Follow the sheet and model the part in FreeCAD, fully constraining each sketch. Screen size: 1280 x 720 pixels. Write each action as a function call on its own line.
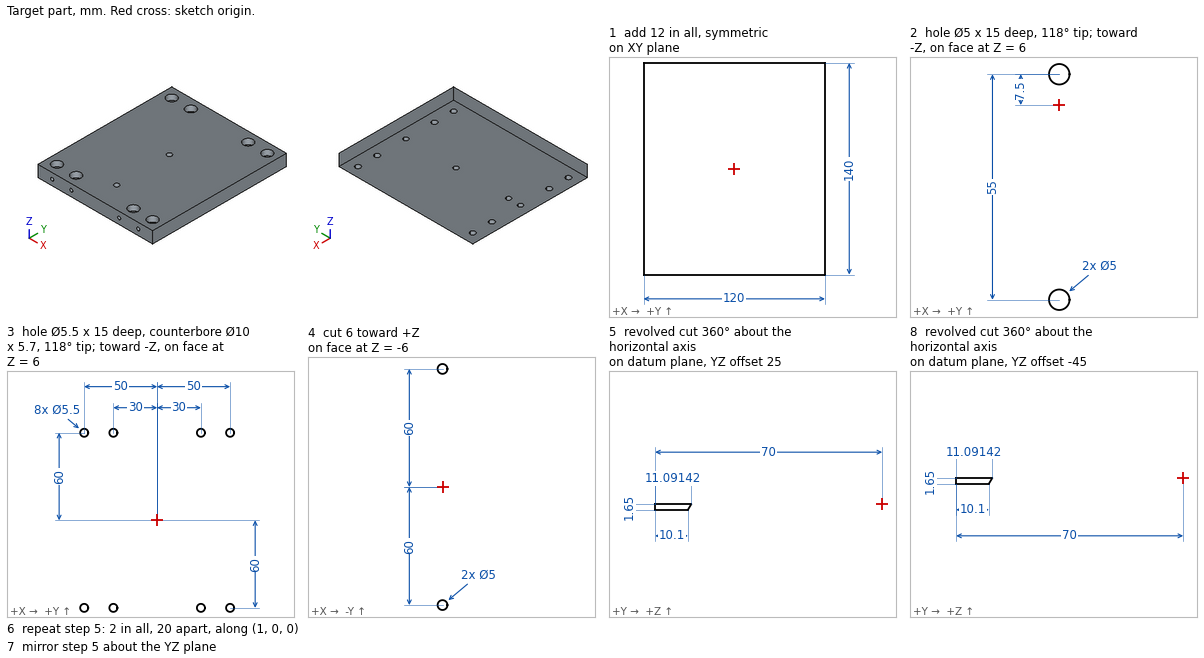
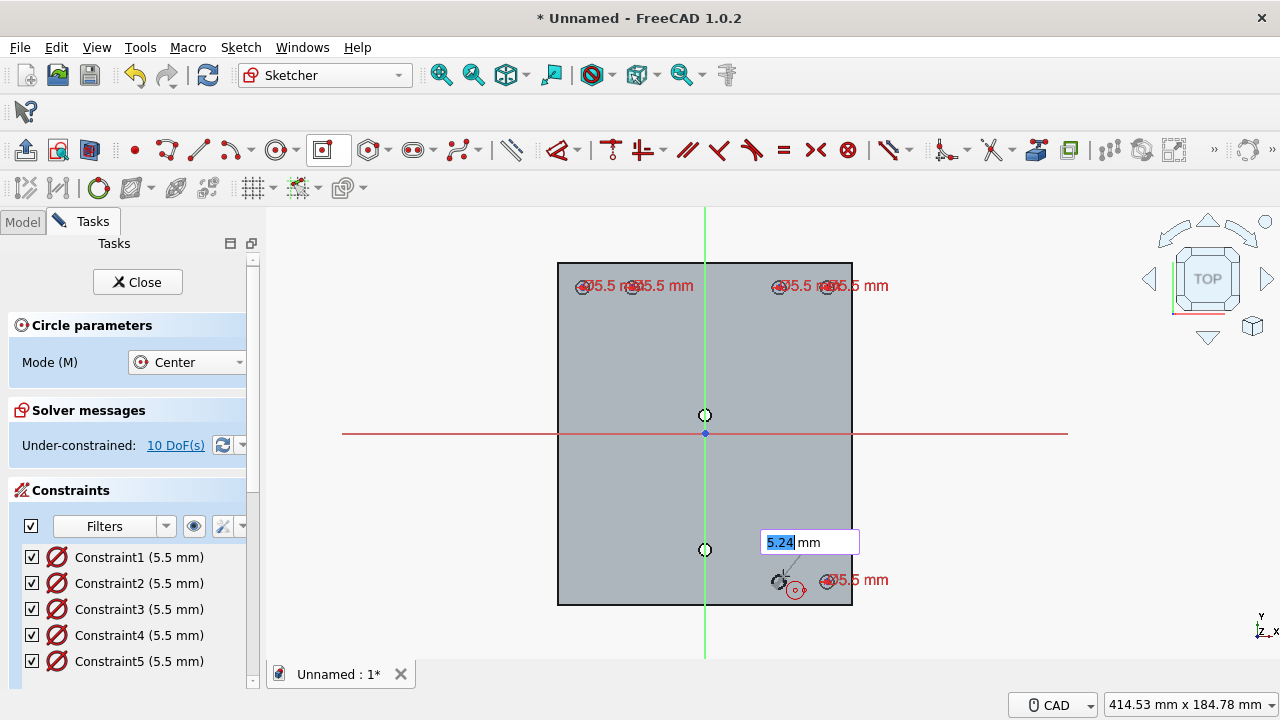
text(5.5)
key(Return)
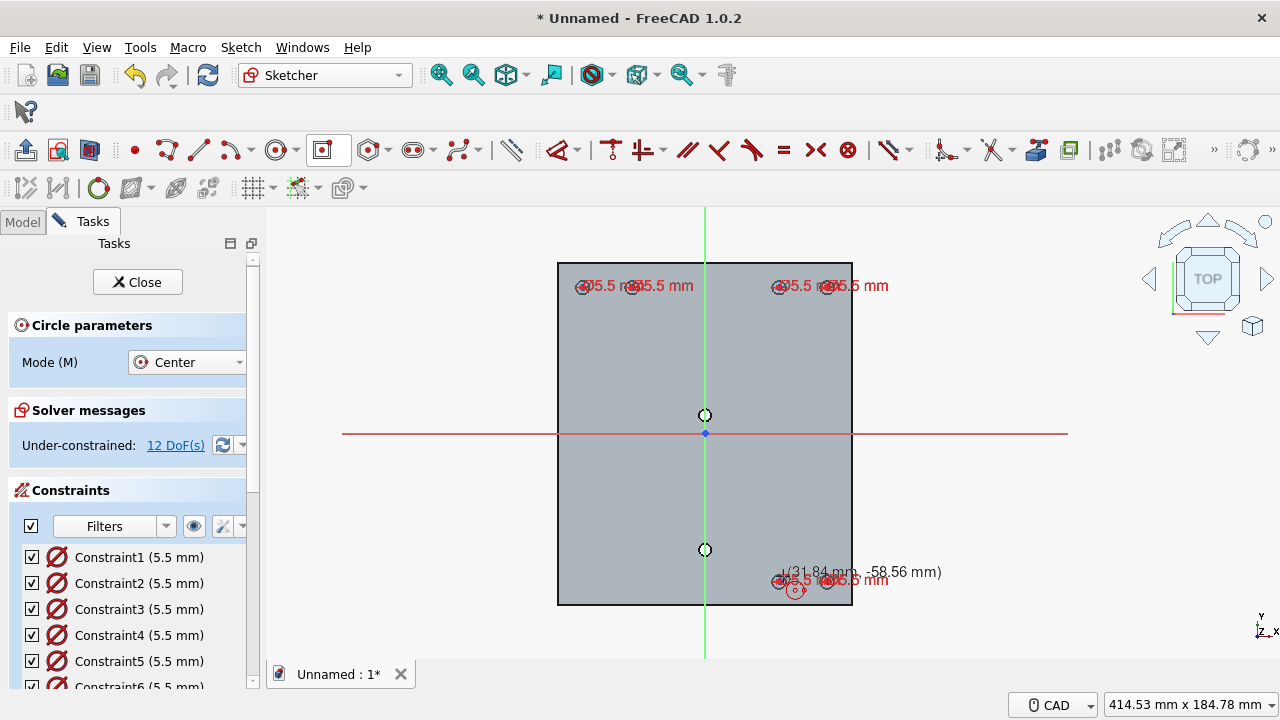
scroll(632, 581, up, 7)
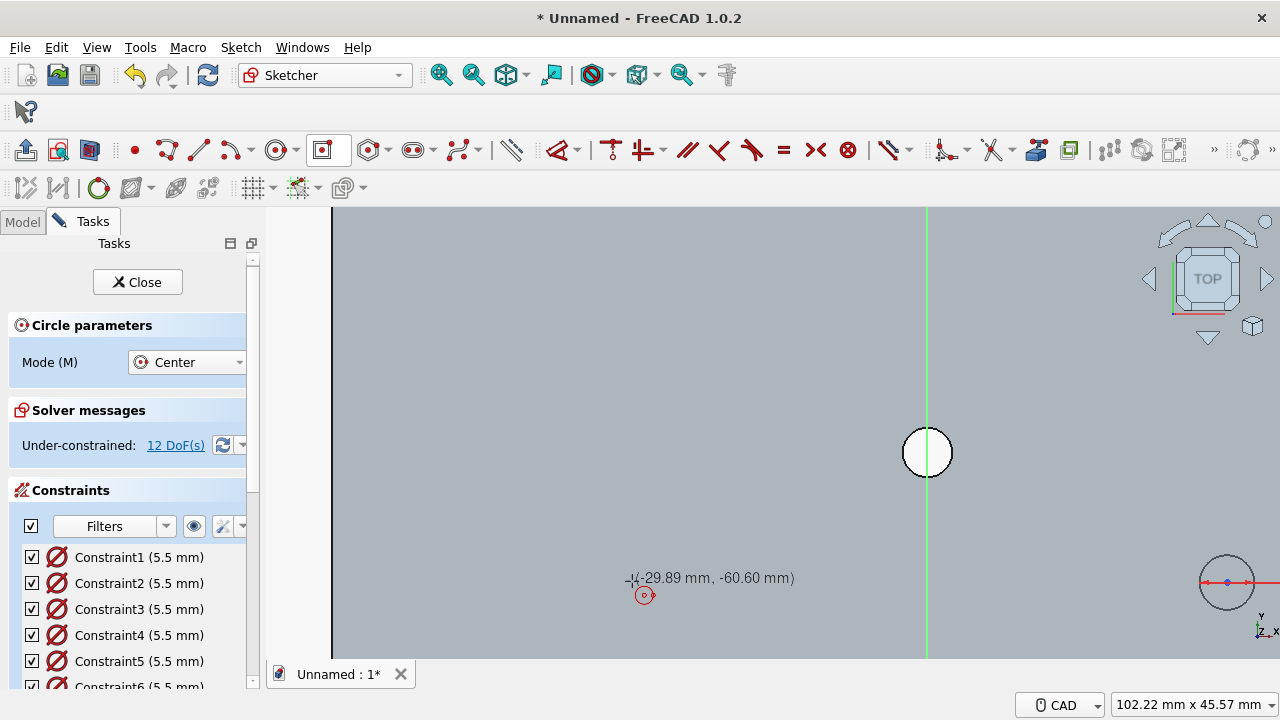
scroll(632, 581, down, 7)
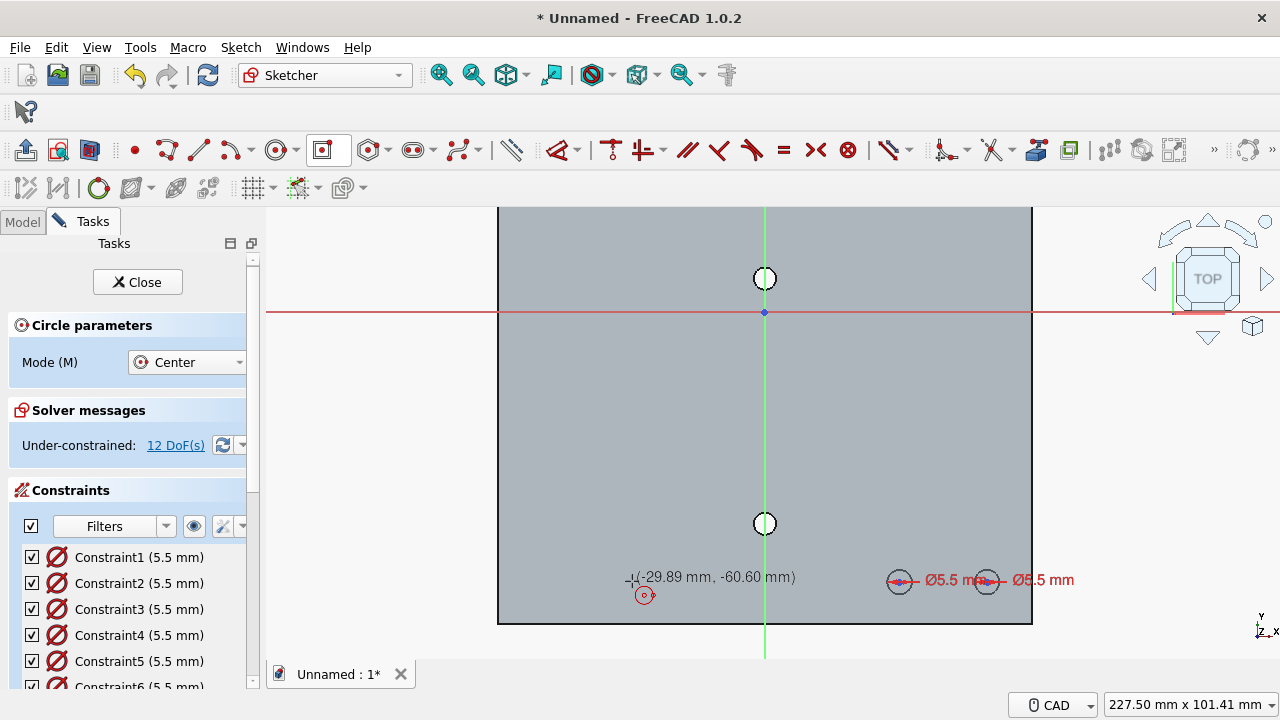
click(632, 581)
move(636, 576)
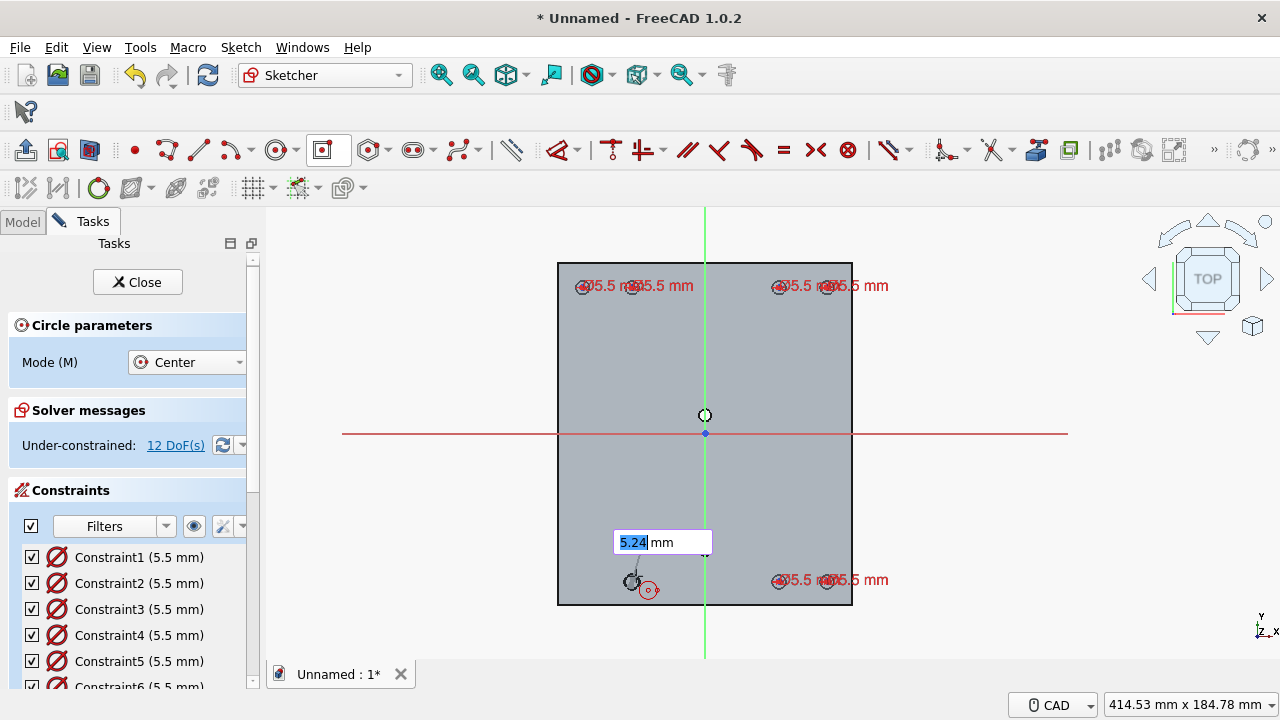
text(5.5)
key(Return)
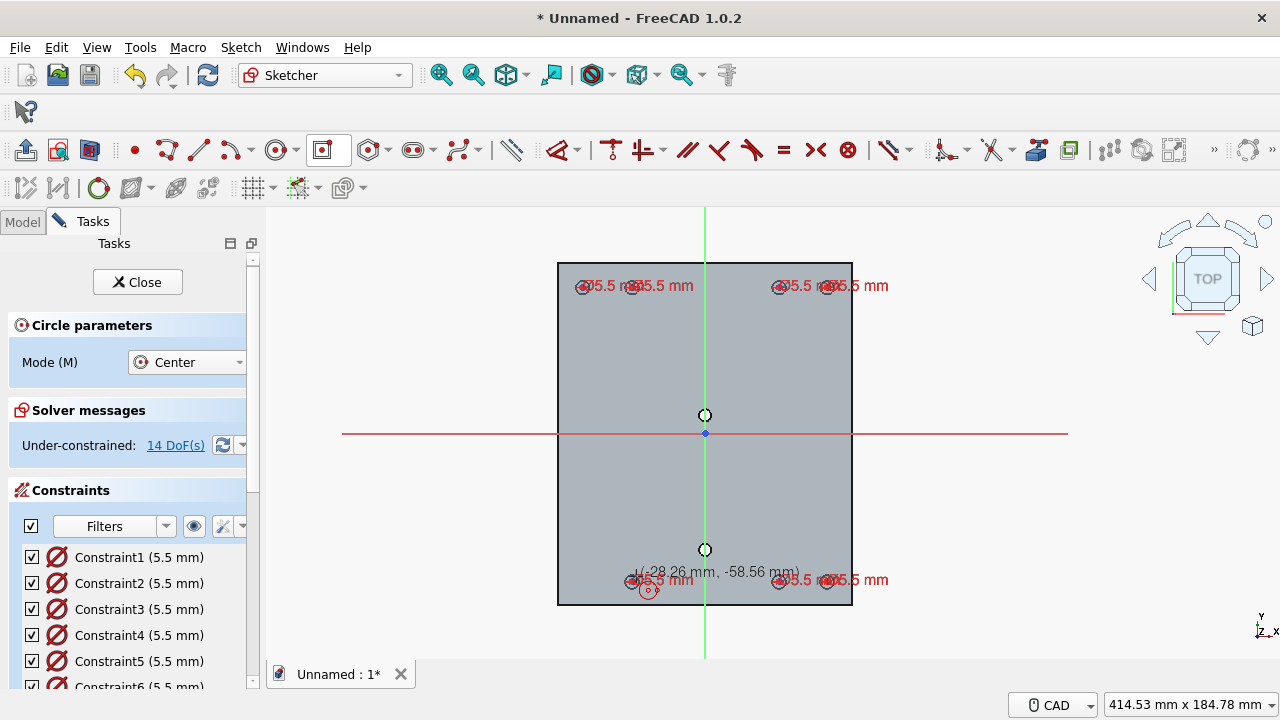
scroll(583, 581, up, 7)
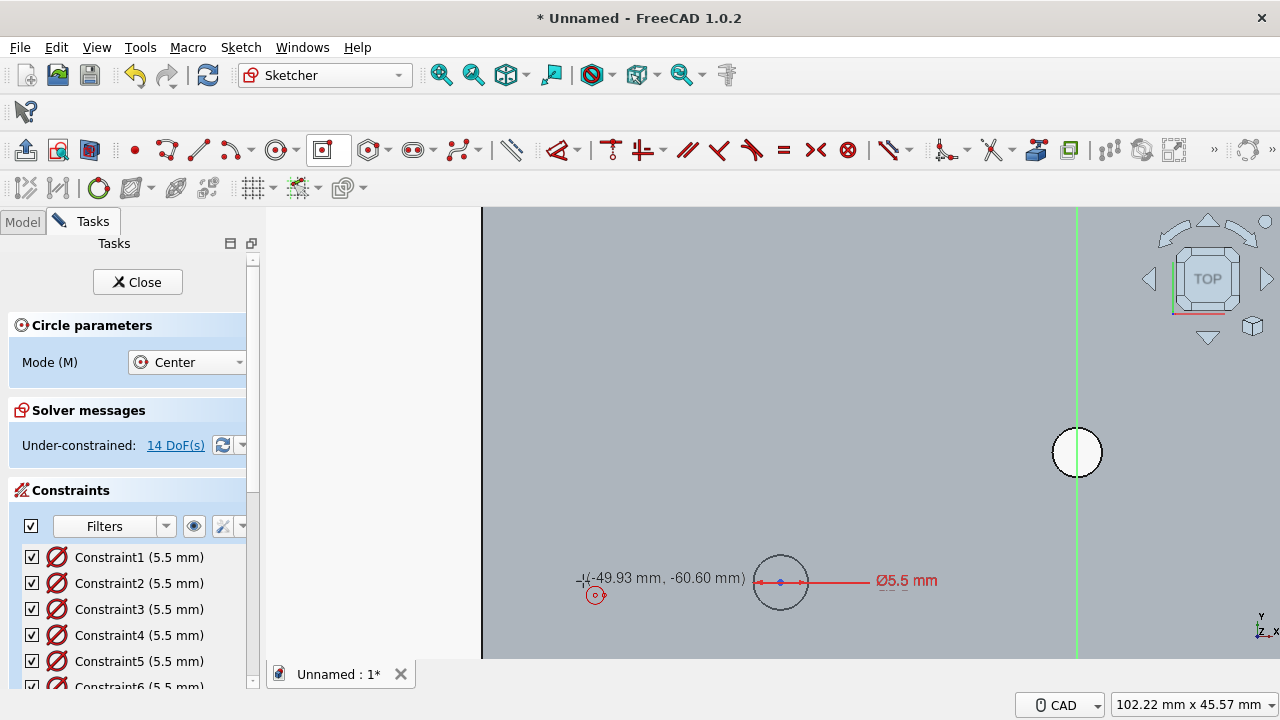
scroll(582, 581, down, 7)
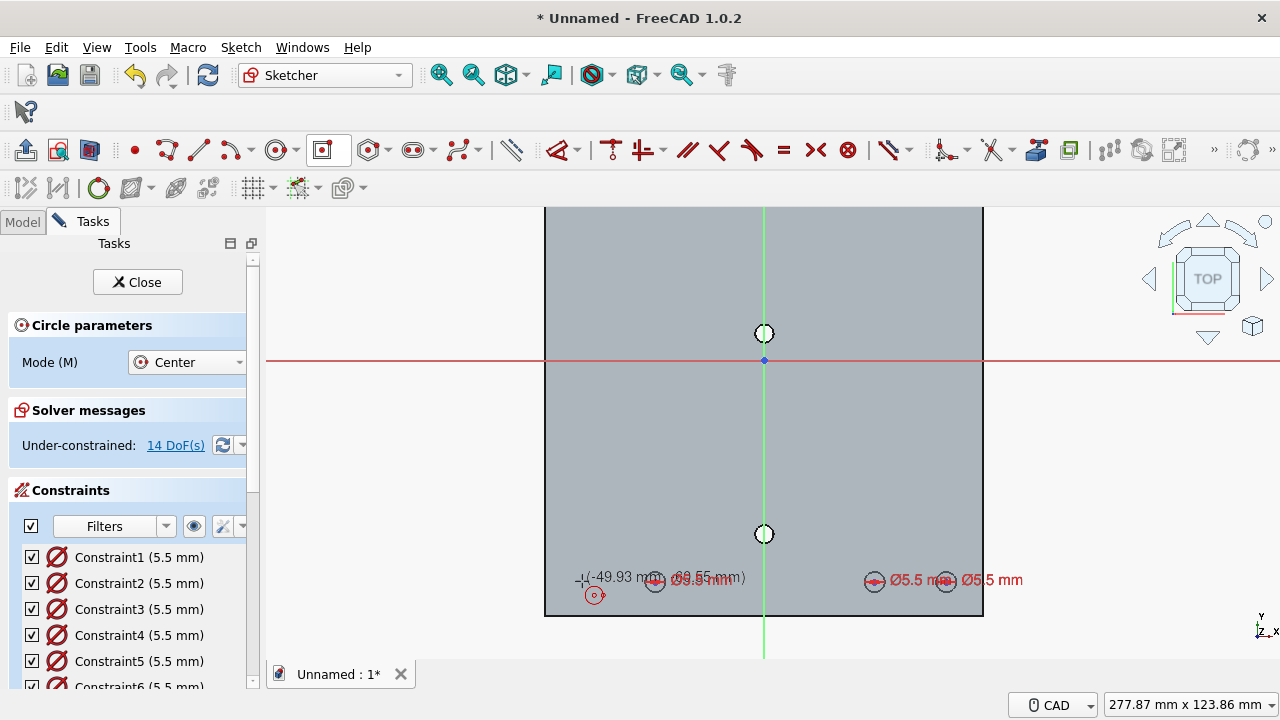
click(582, 581)
move(587, 576)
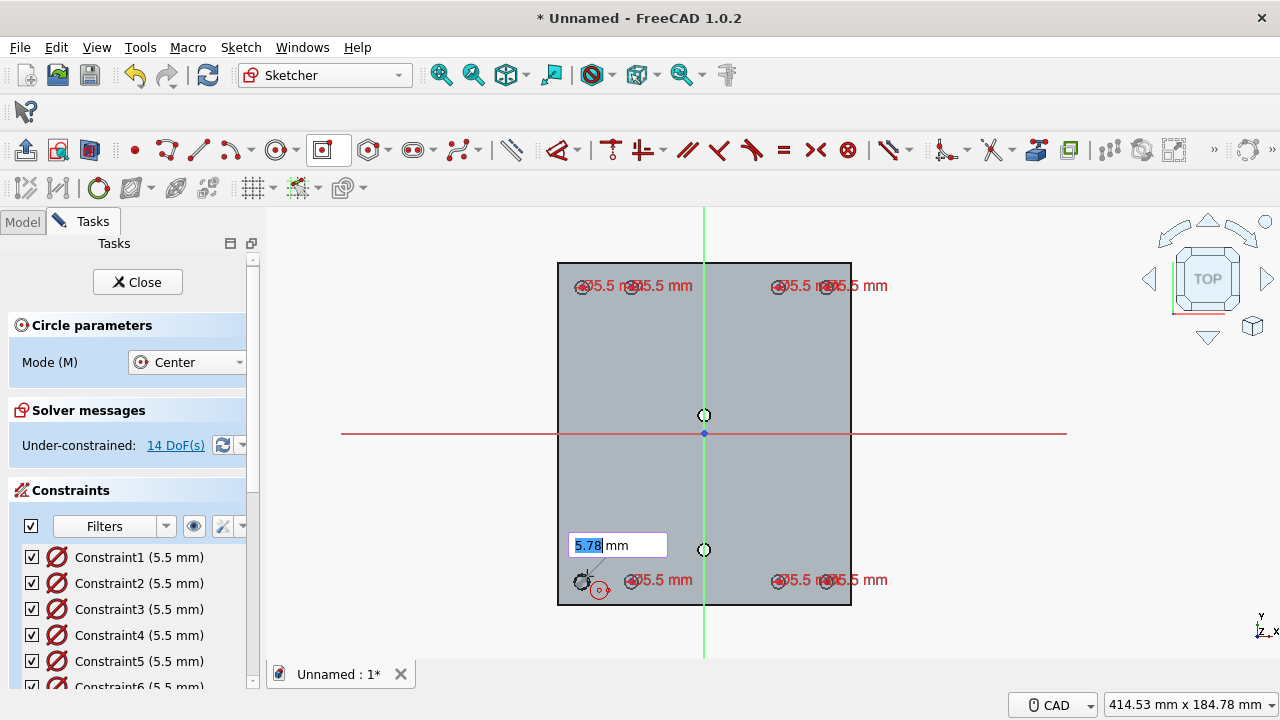
text(5.5)
key(Return)
key(Escape)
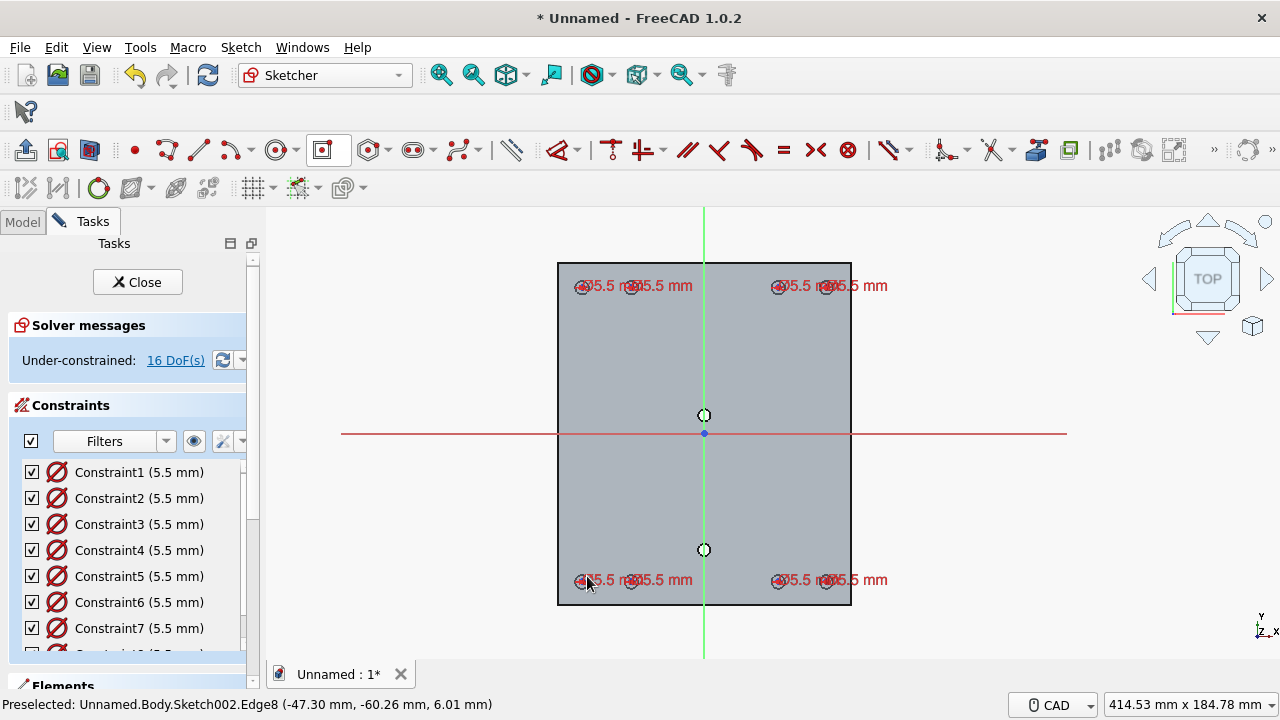
click(582, 288)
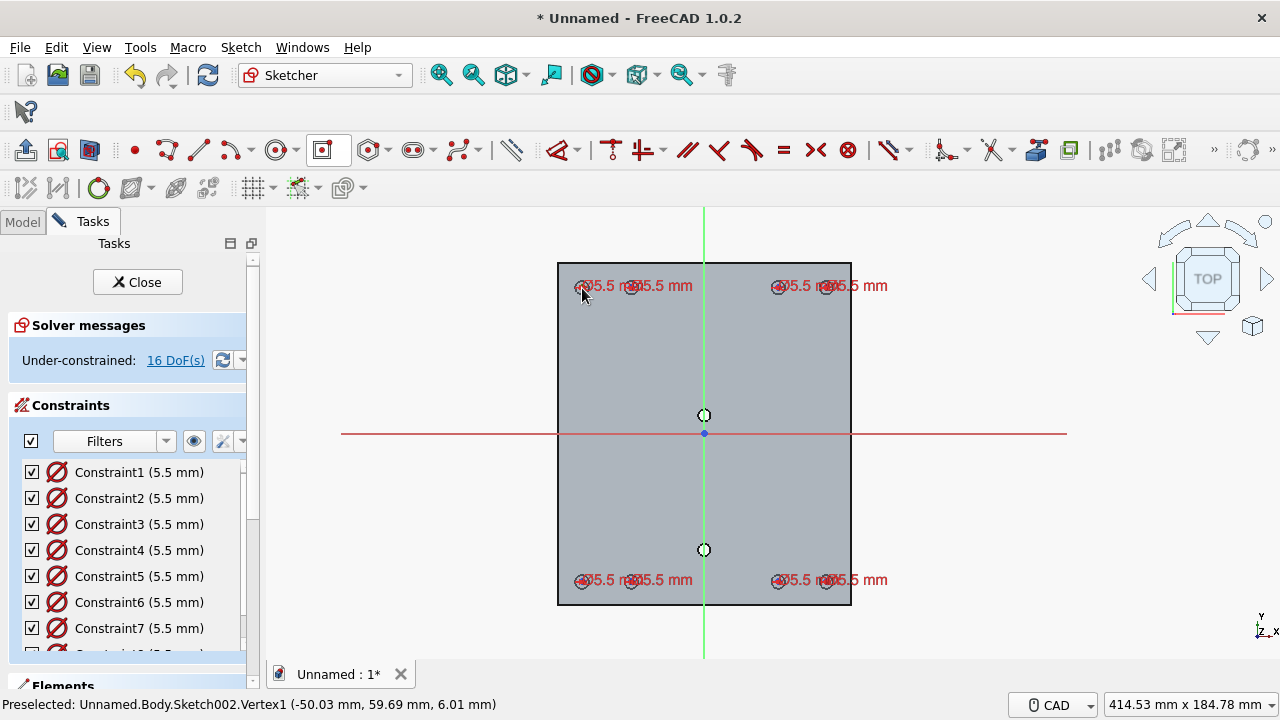
click(631, 288)